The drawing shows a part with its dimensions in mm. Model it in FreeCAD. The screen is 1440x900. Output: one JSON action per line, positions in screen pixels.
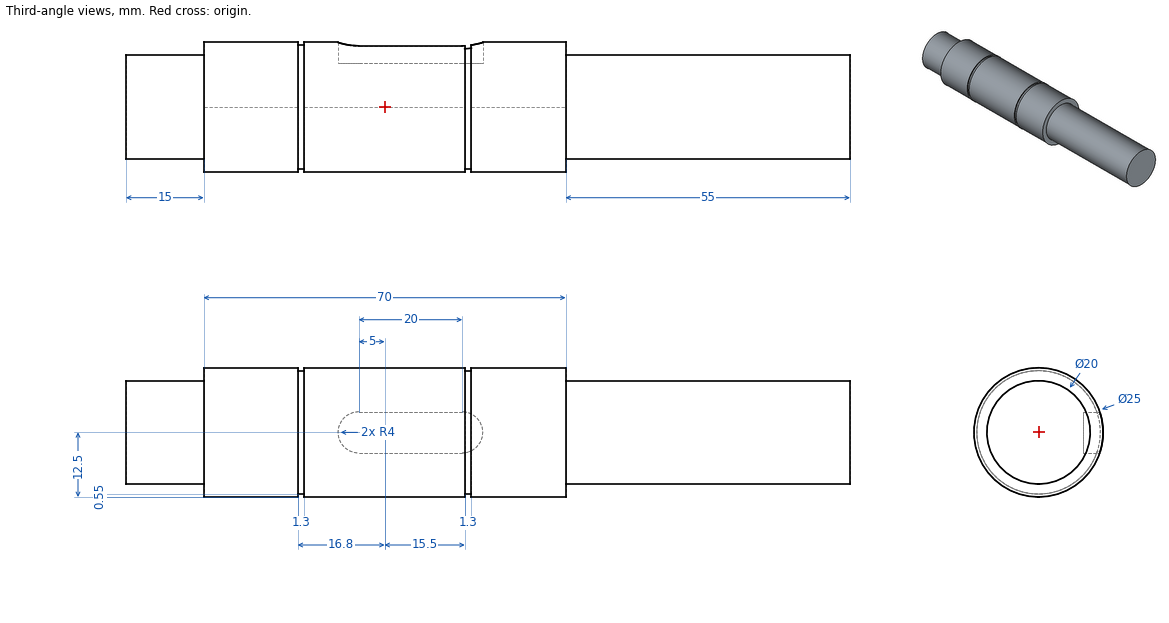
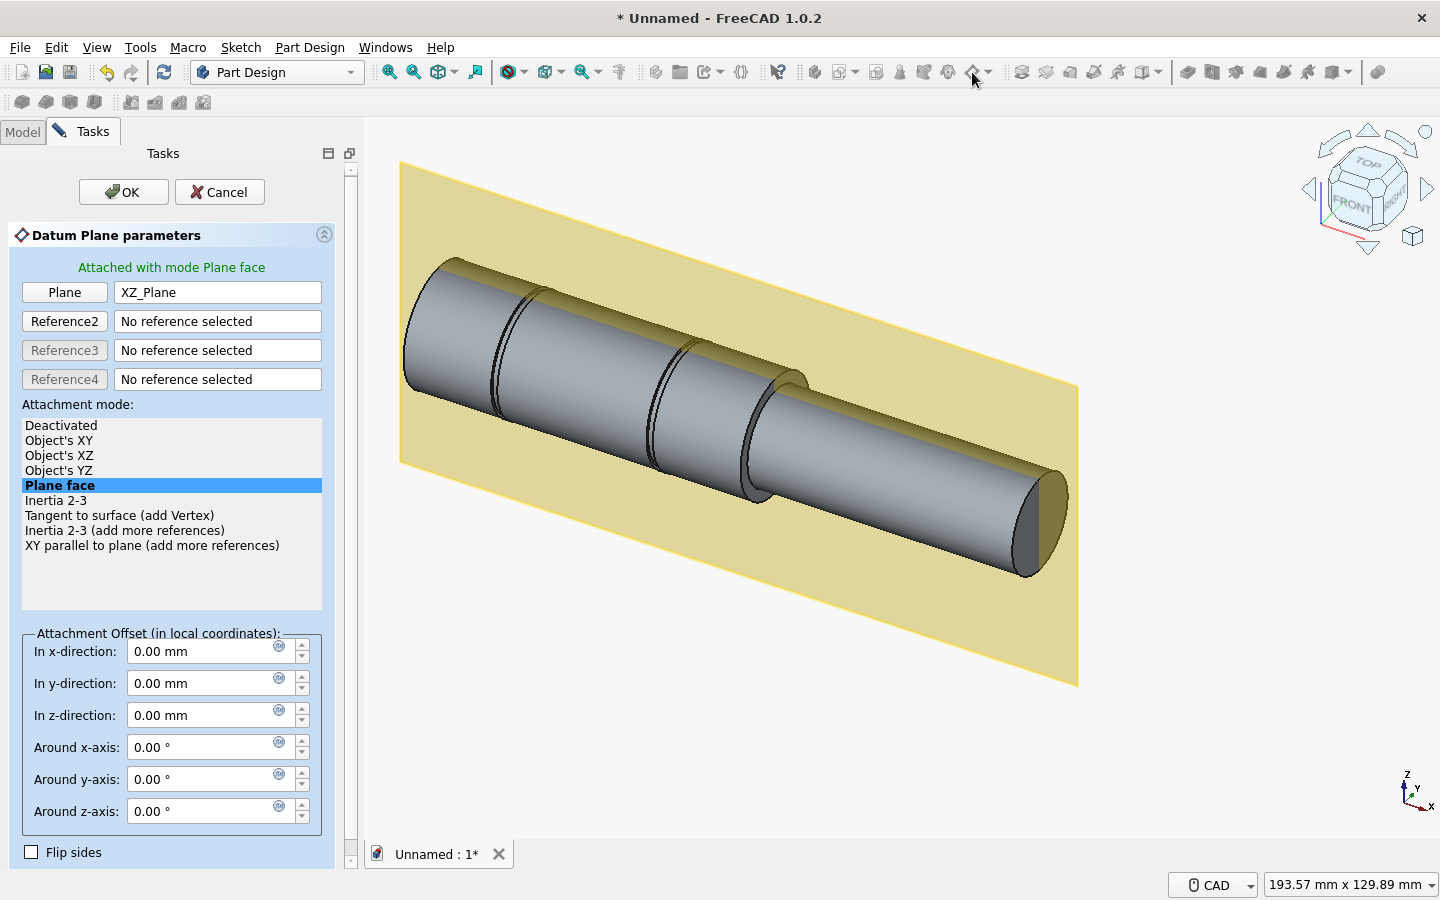
{"action": "triple_click", "coordinate": [210, 715]}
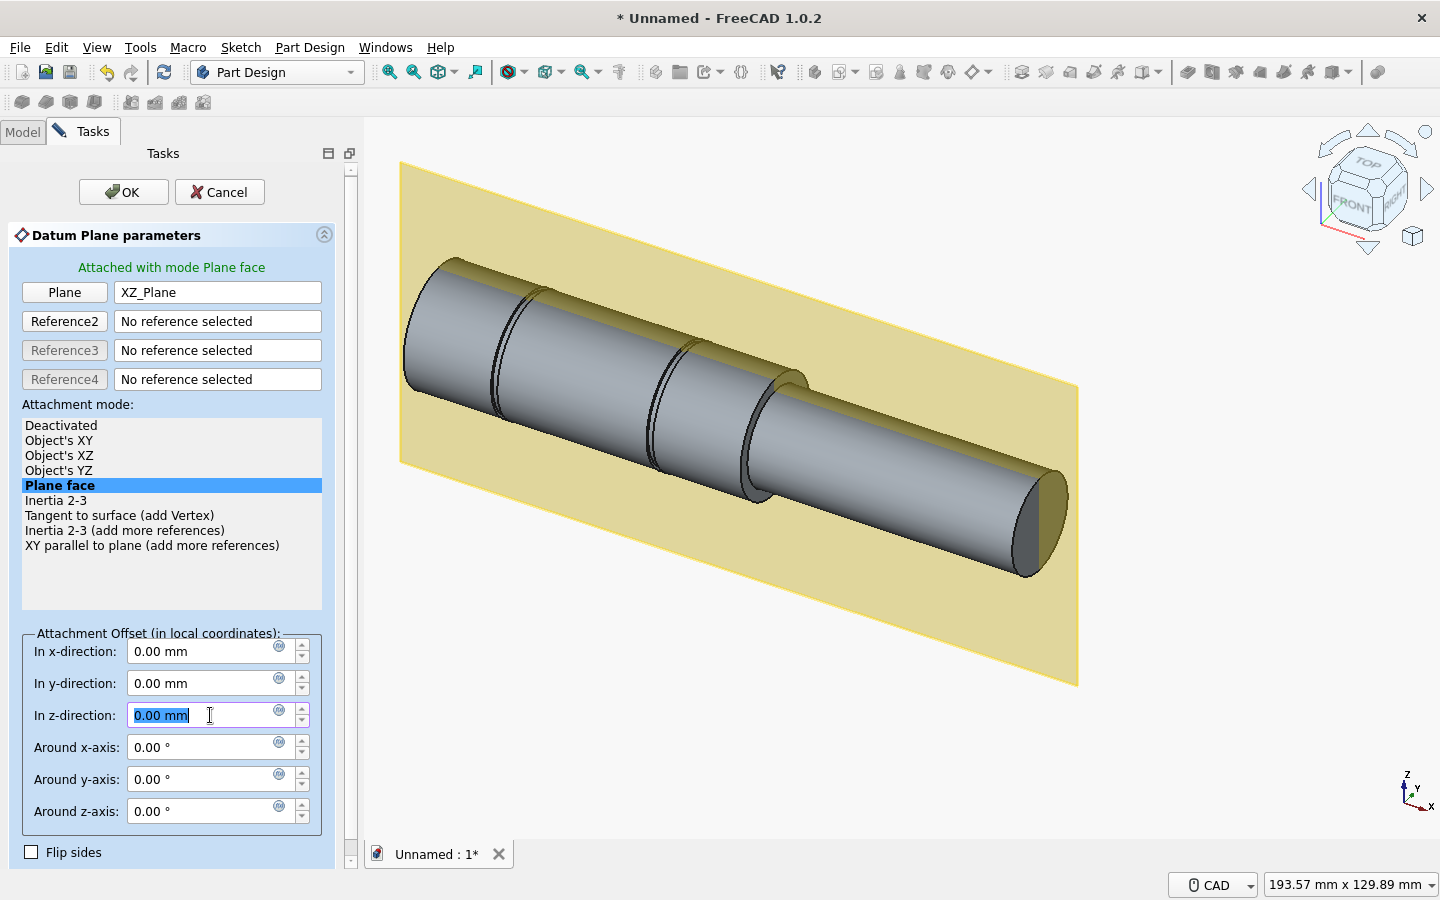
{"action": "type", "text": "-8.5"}
{"action": "key", "text": "Tab"}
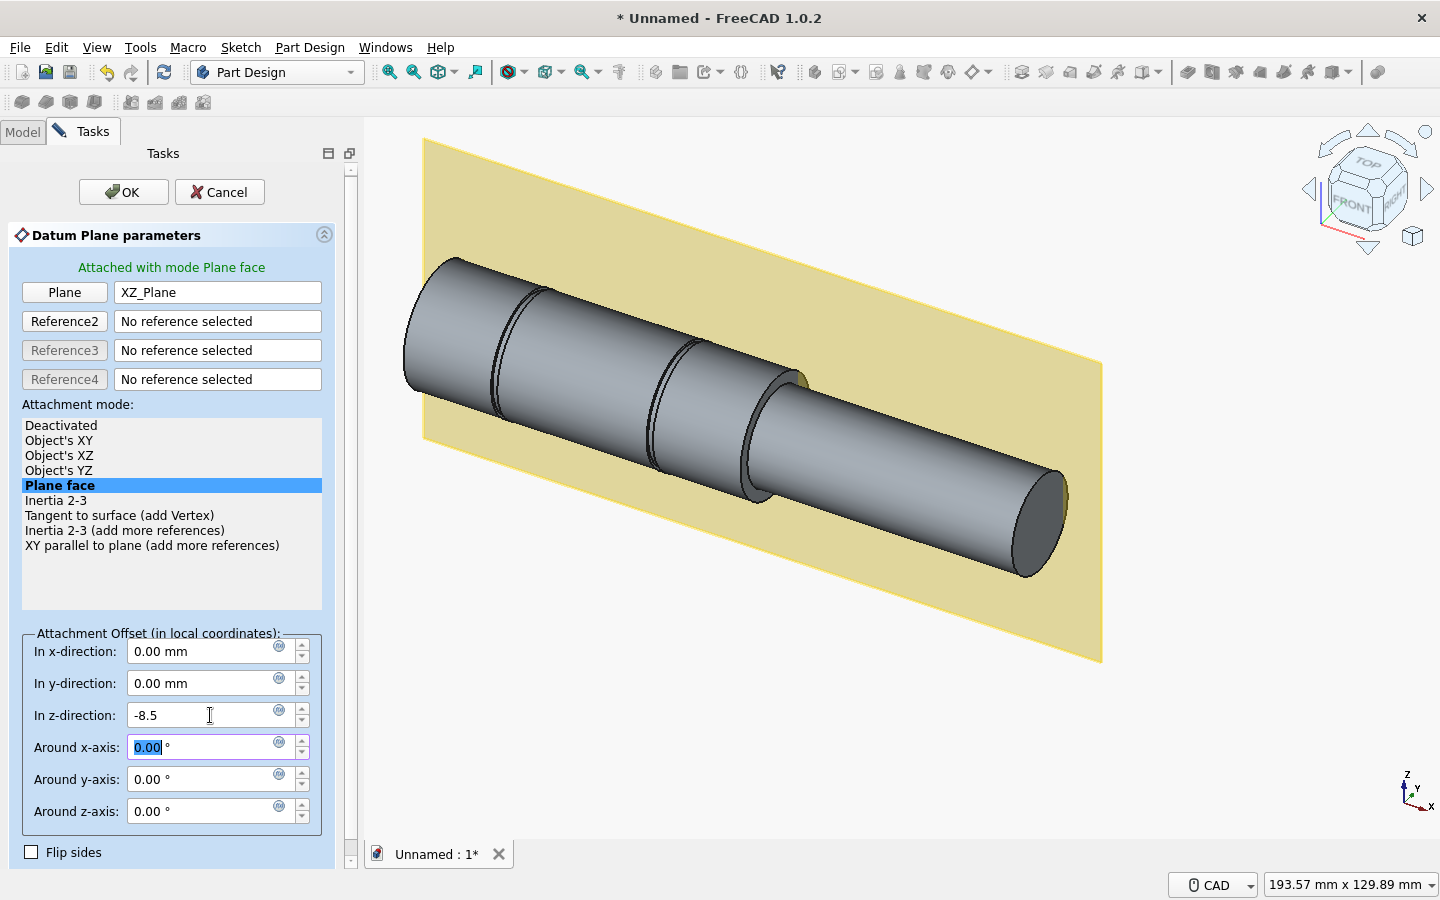
{"action": "left_click", "coordinate": [124, 192]}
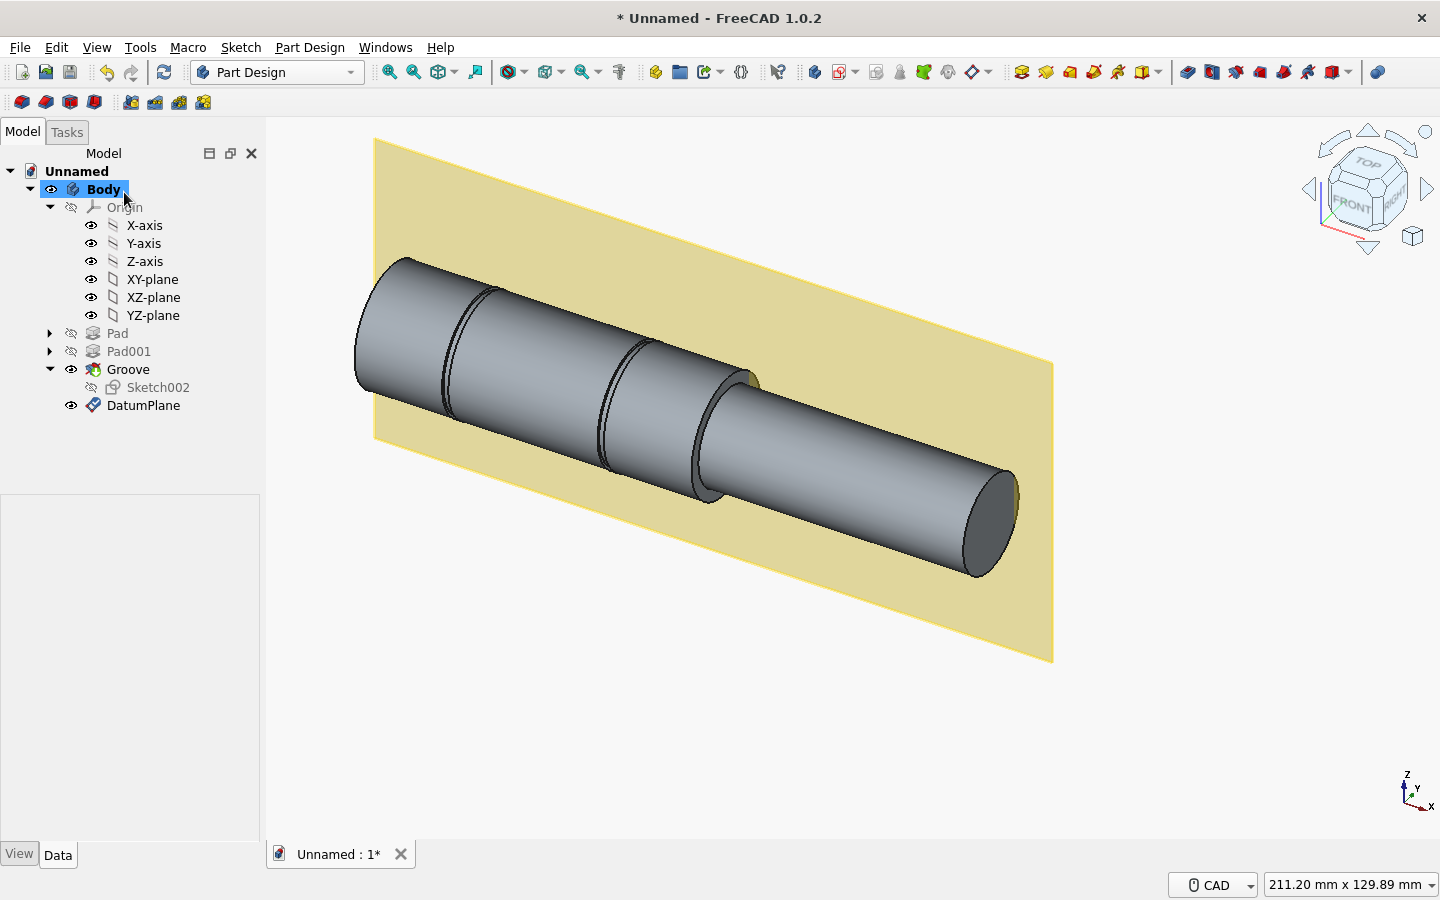
{"action": "left_click", "coordinate": [116, 405]}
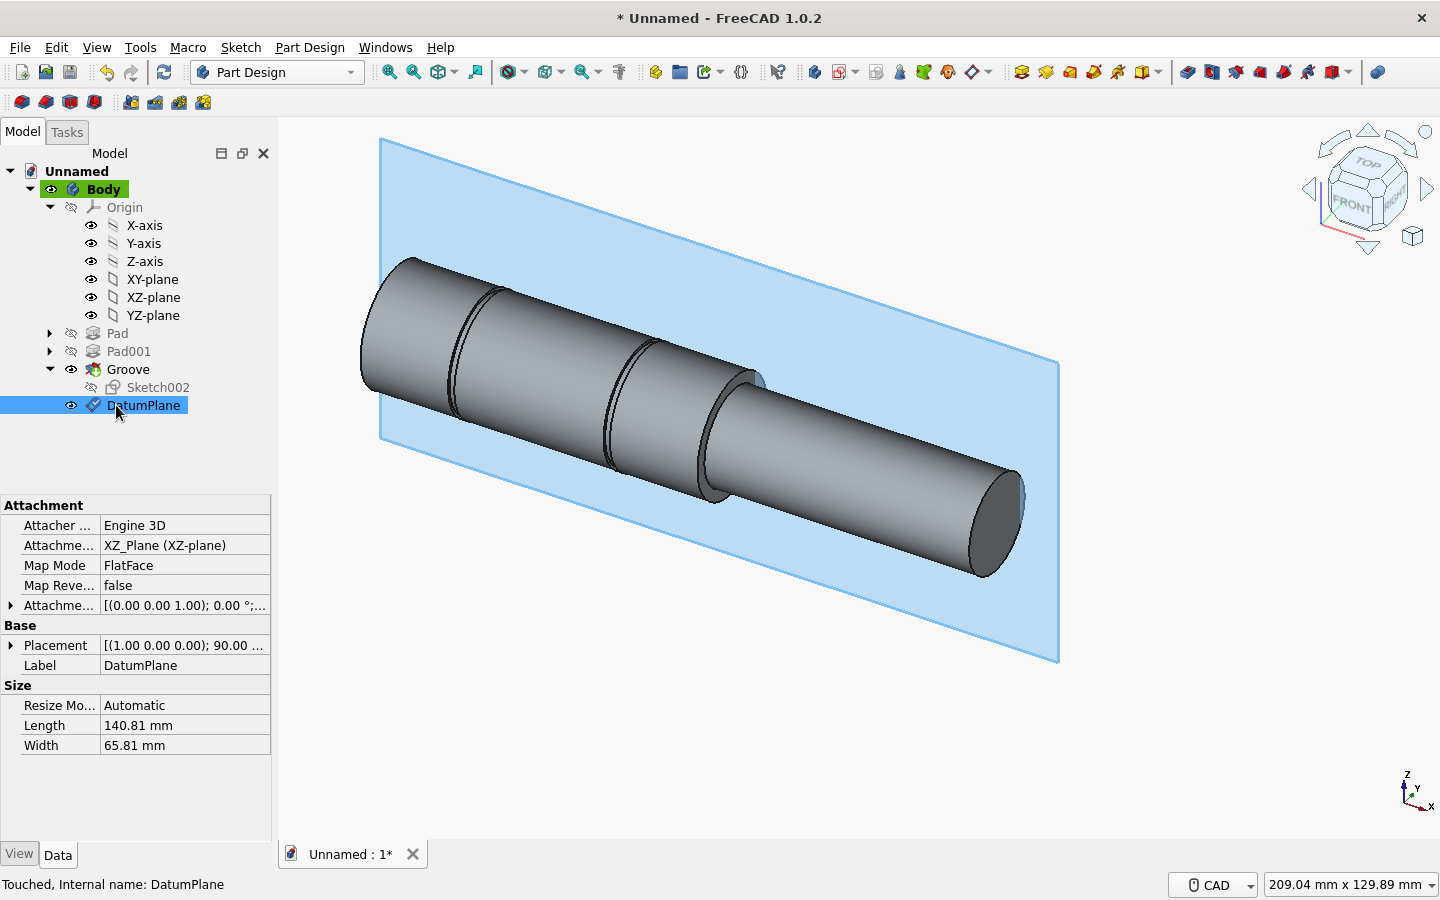
{"action": "left_click", "coordinate": [840, 72]}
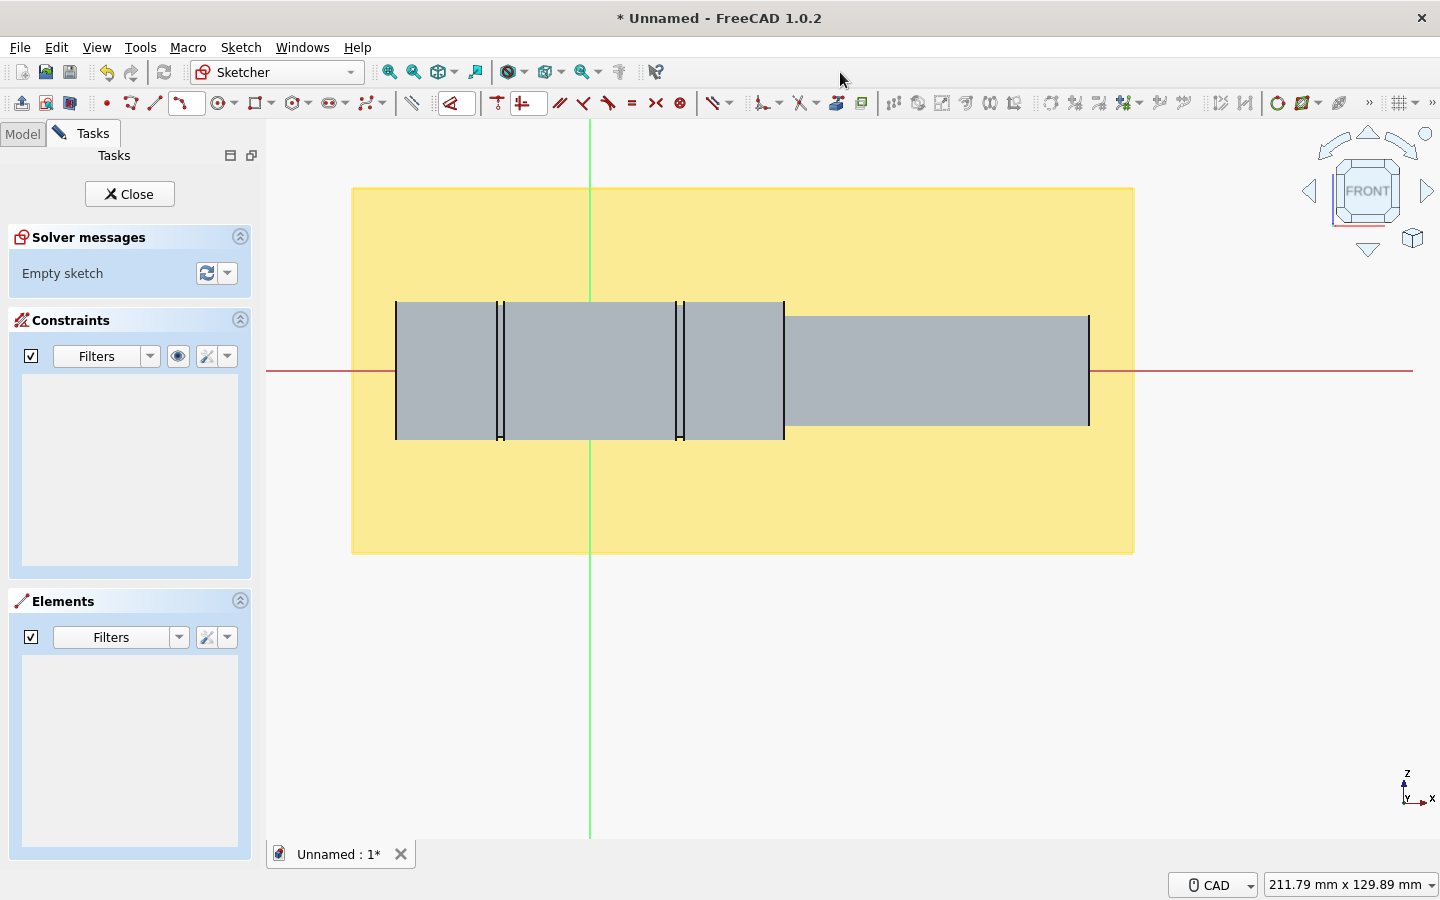
{"action": "left_click", "coordinate": [70, 104]}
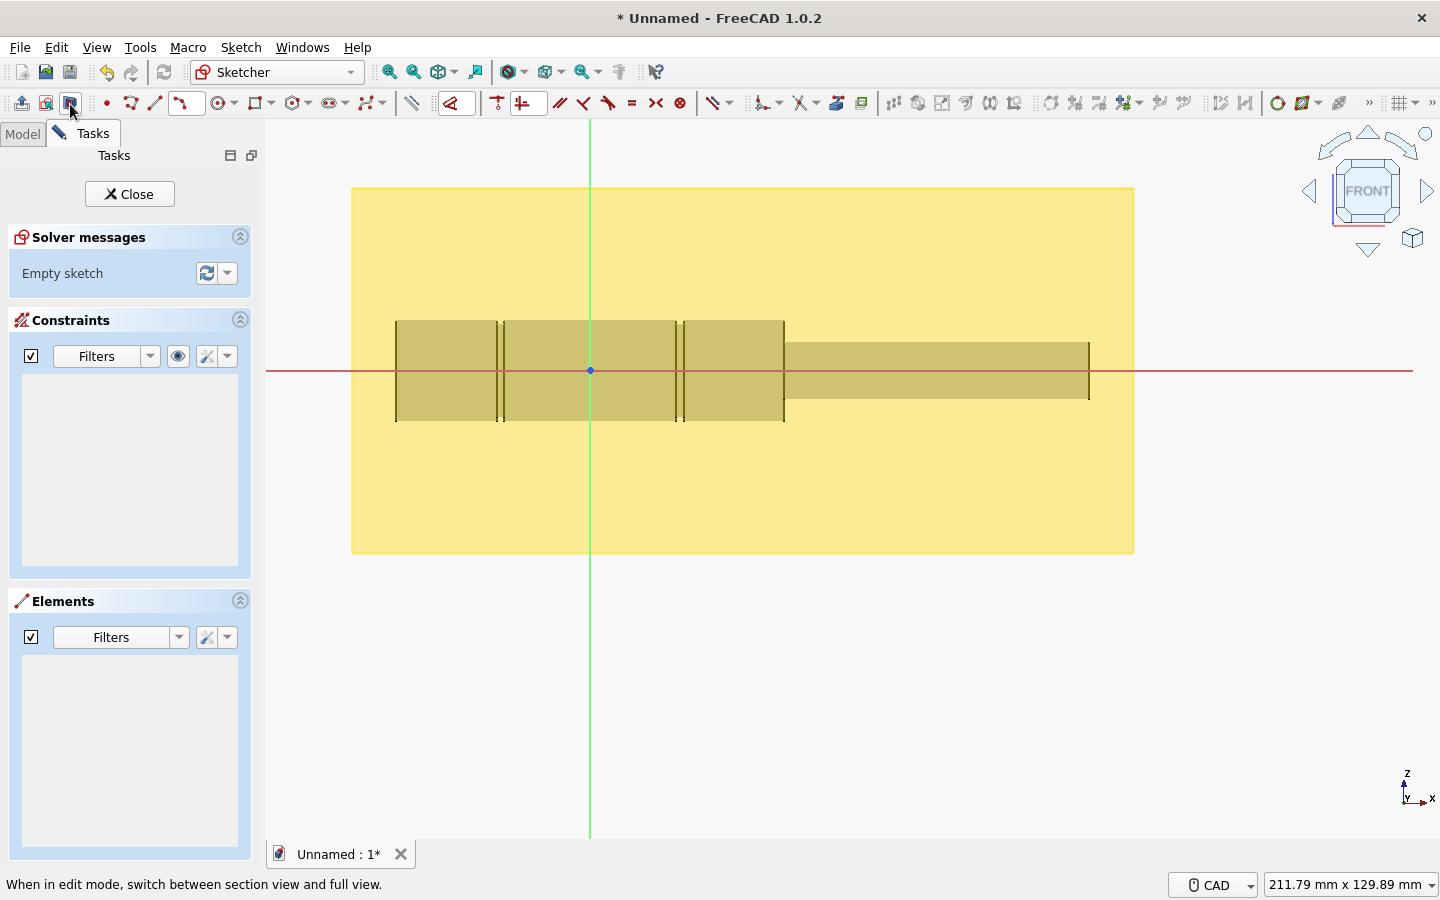
{"action": "scroll", "coordinate": [564, 335], "scroll_direction": "up", "scroll_amount": 7}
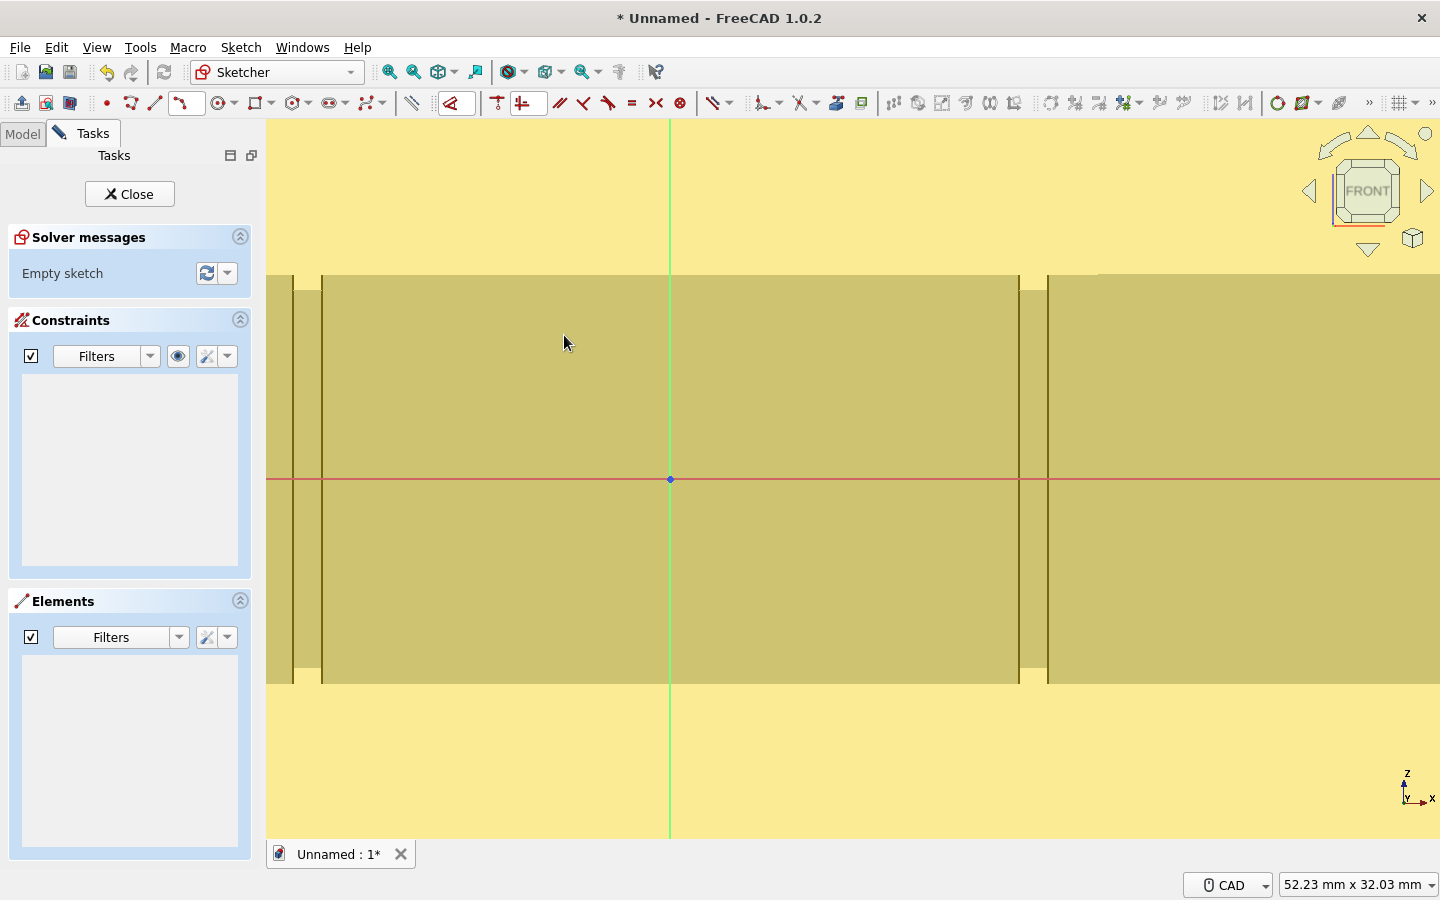
{"action": "left_click", "coordinate": [330, 104]}